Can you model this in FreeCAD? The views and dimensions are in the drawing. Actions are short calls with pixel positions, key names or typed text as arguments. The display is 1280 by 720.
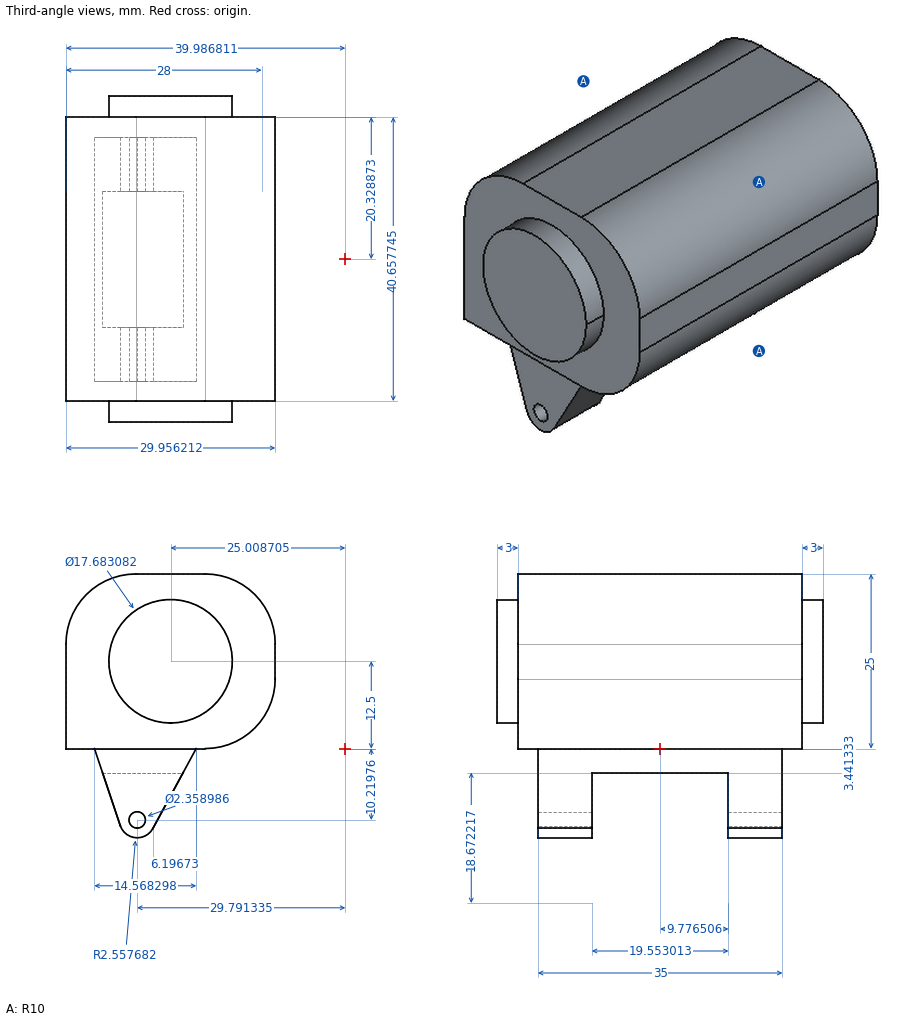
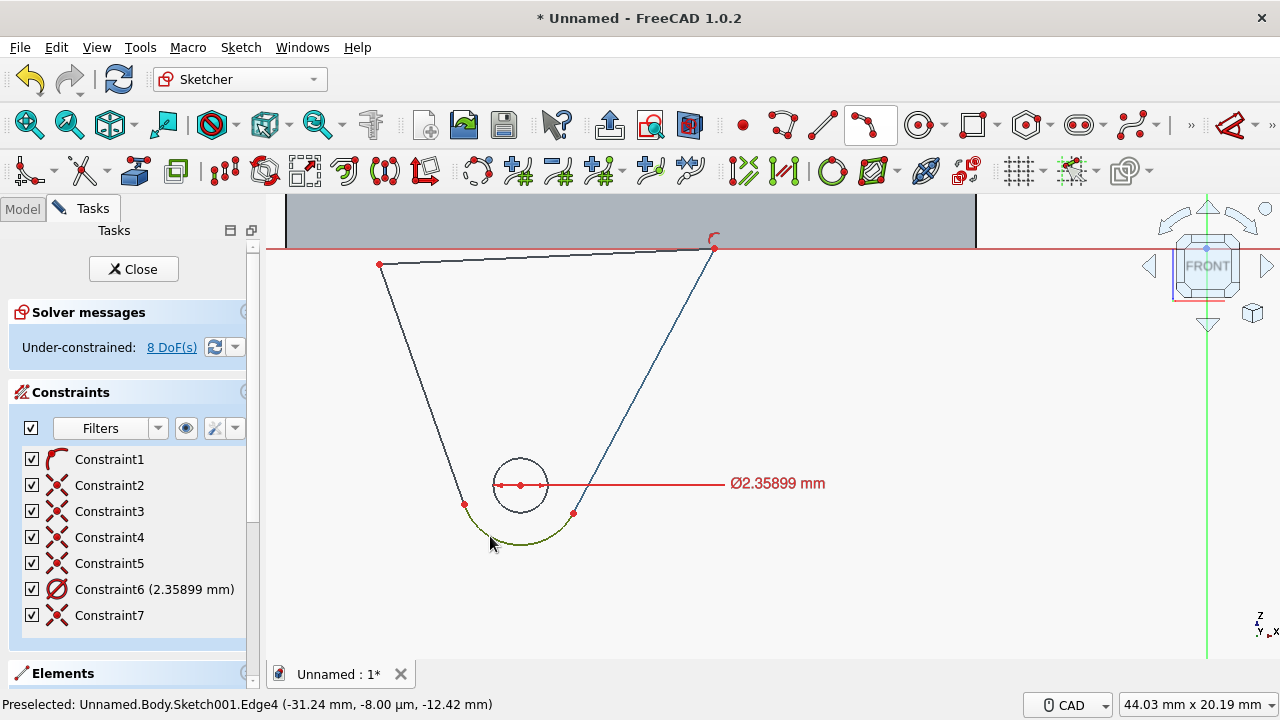
key(t)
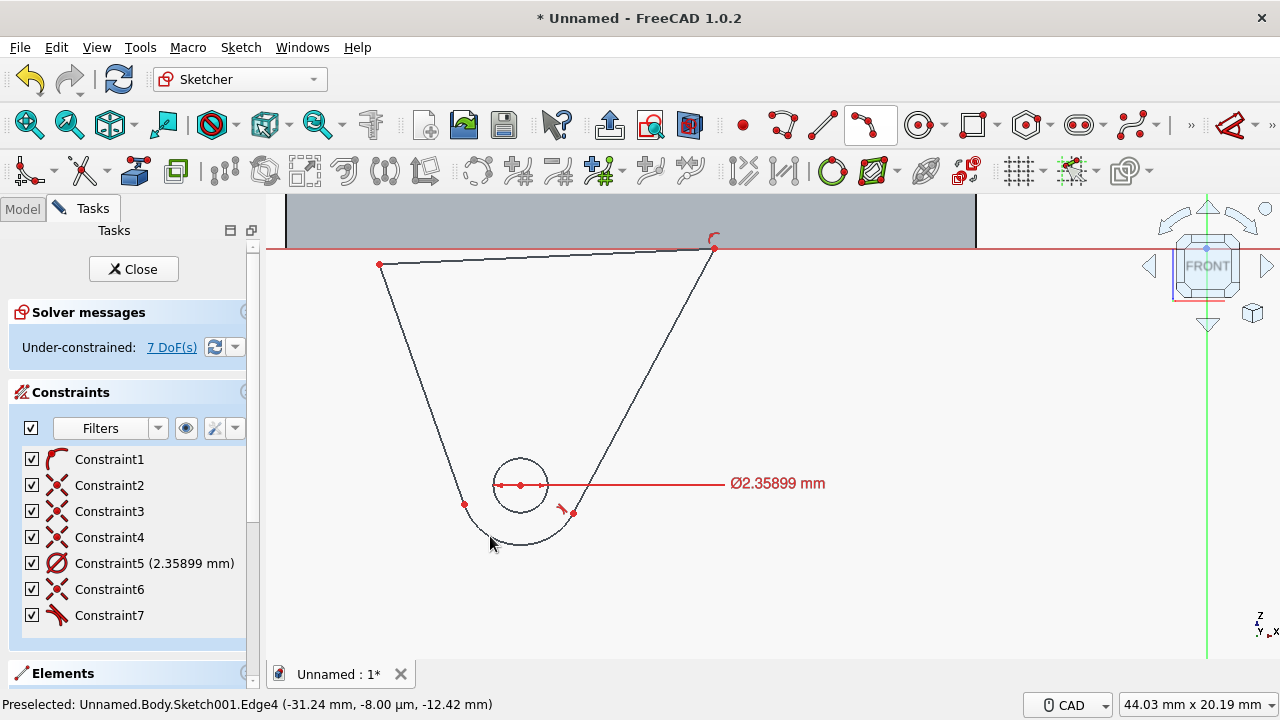
click(405, 336)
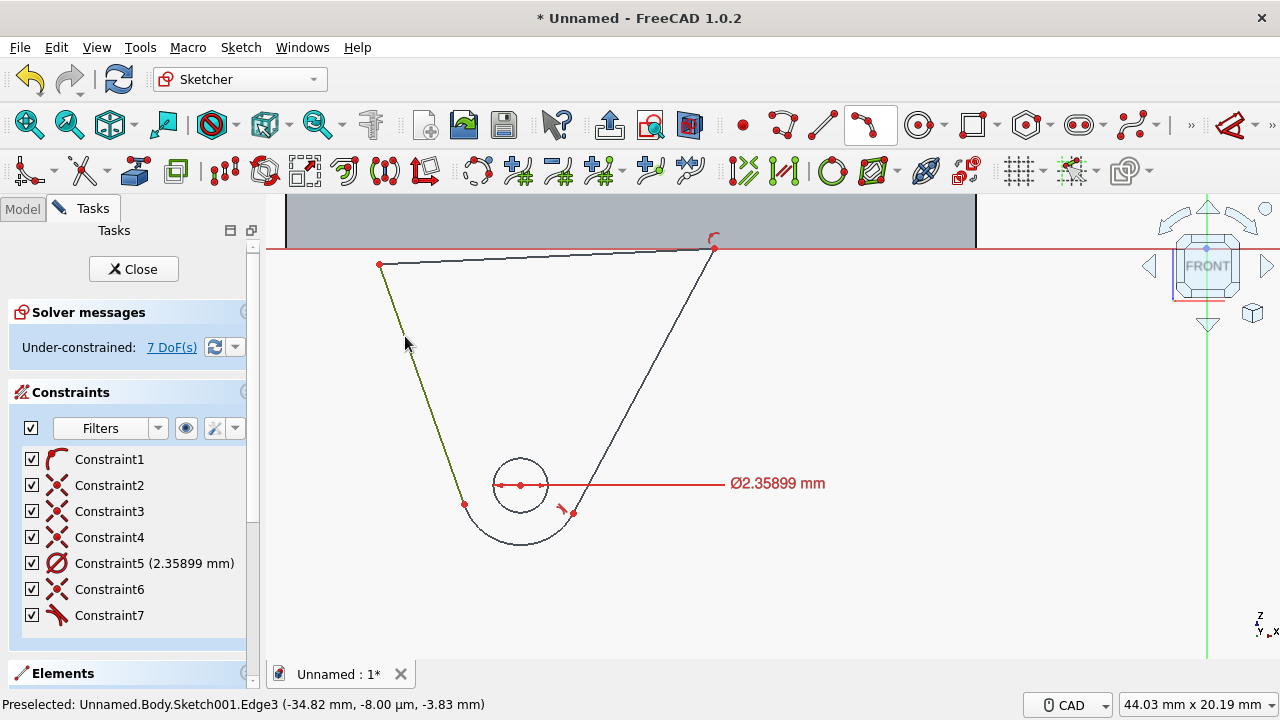
click(490, 536)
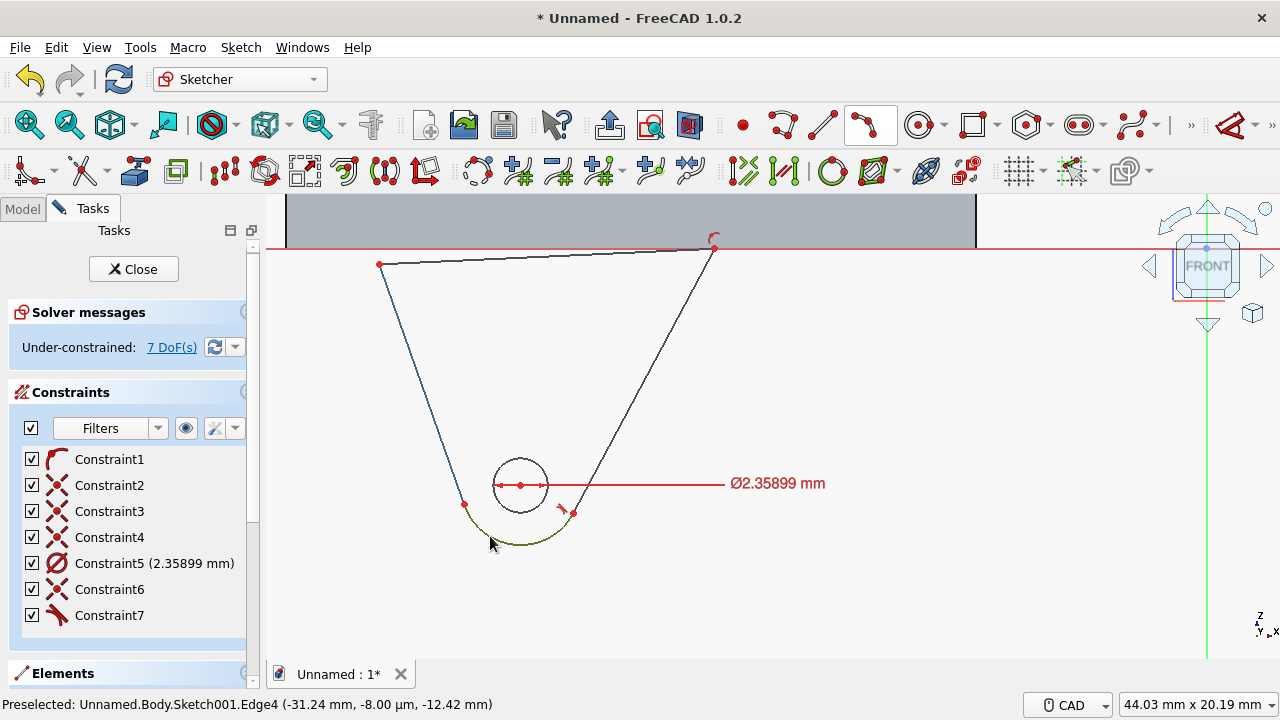
key(t)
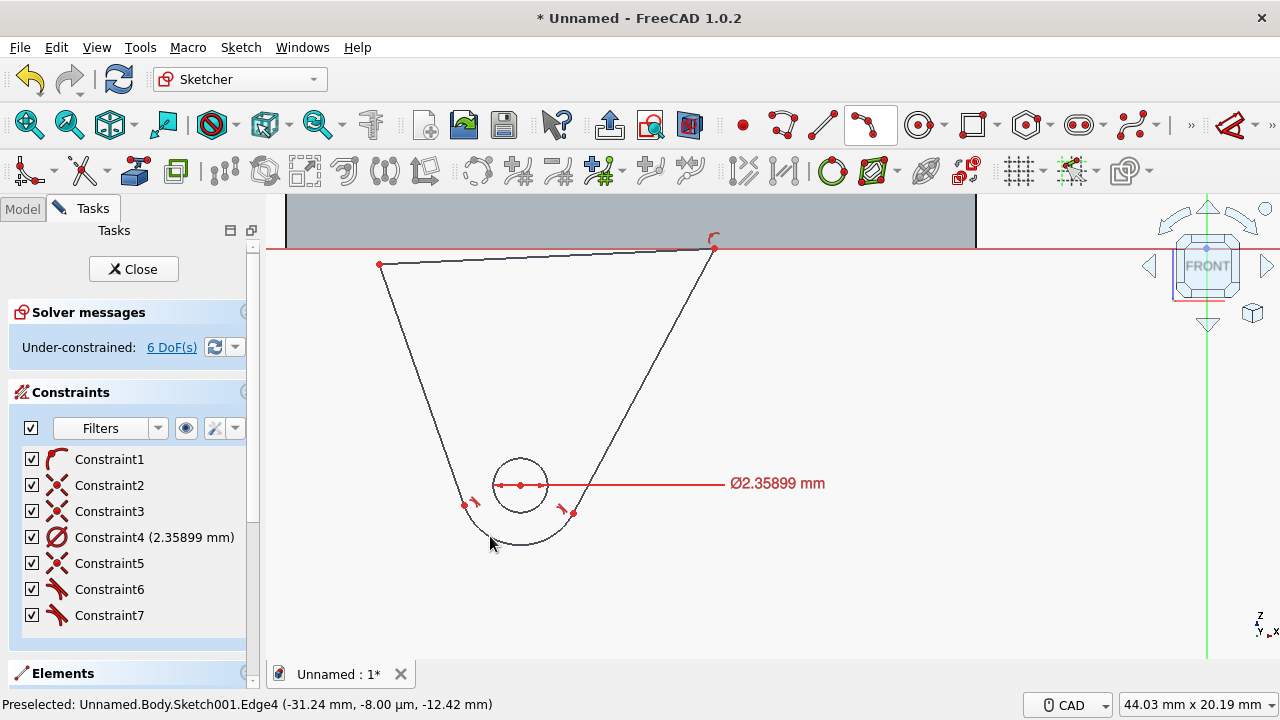
scroll(480, 260, up, 2)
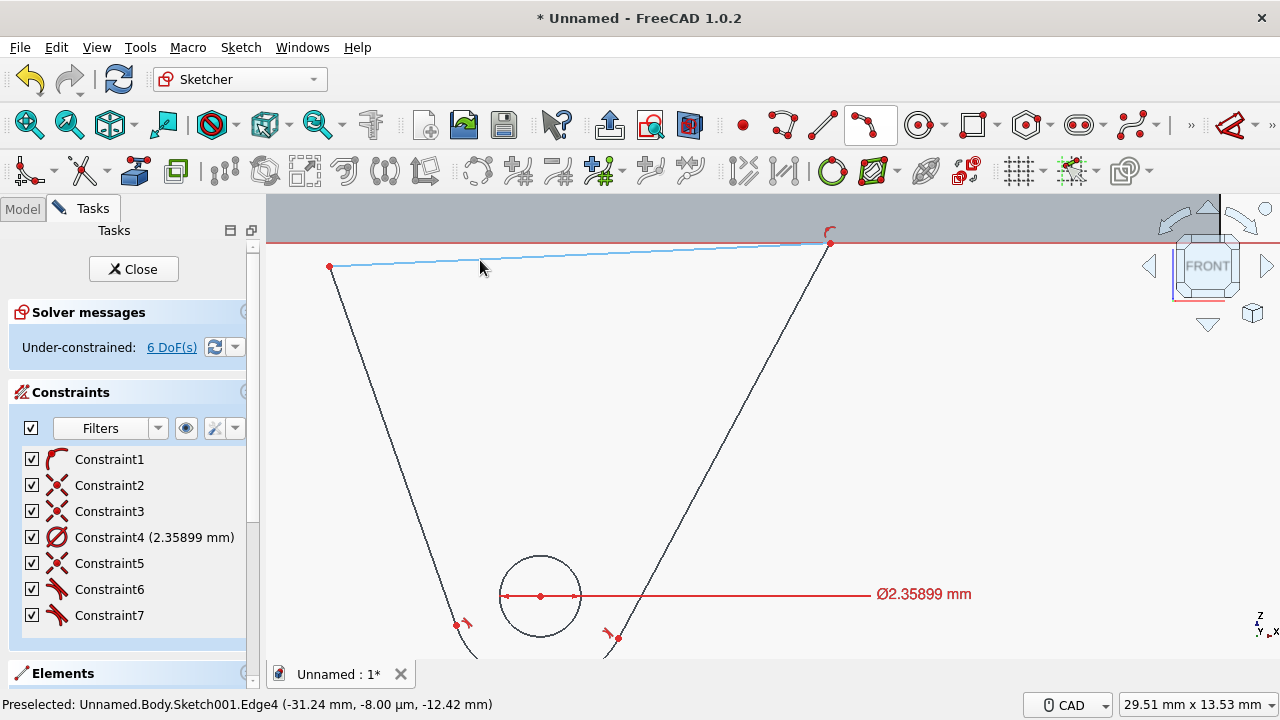
click(480, 259)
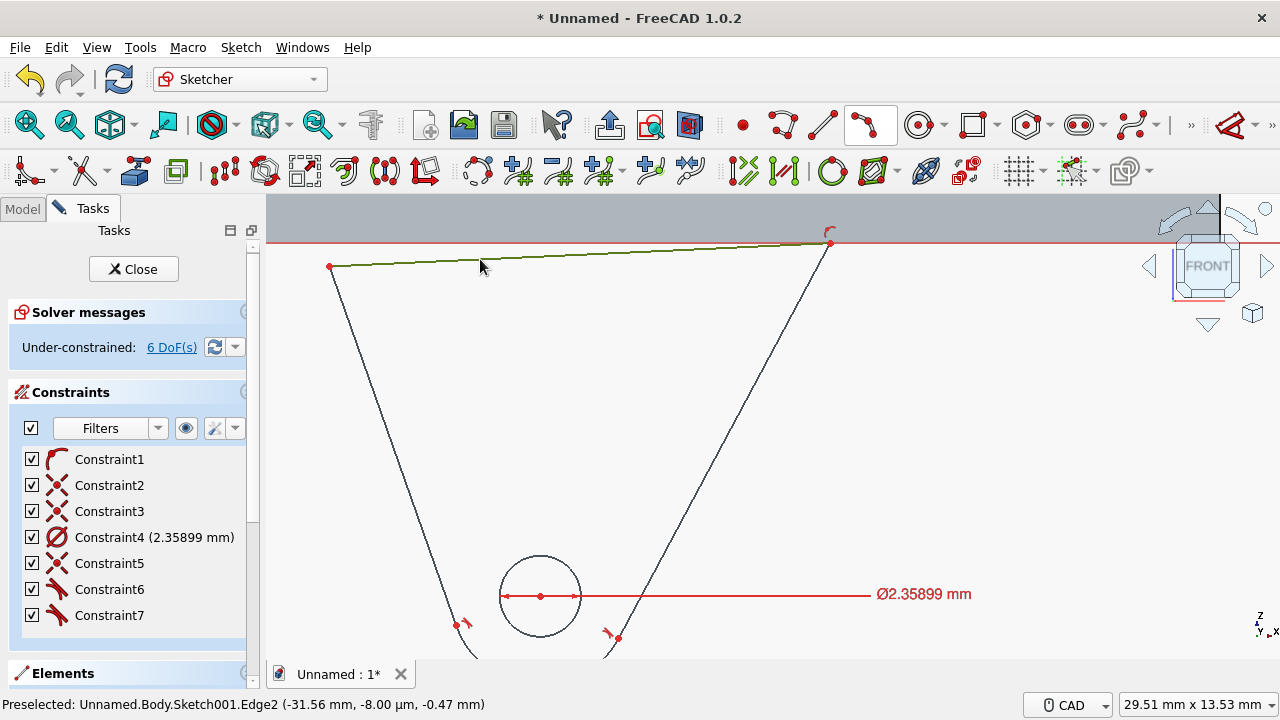
key(h)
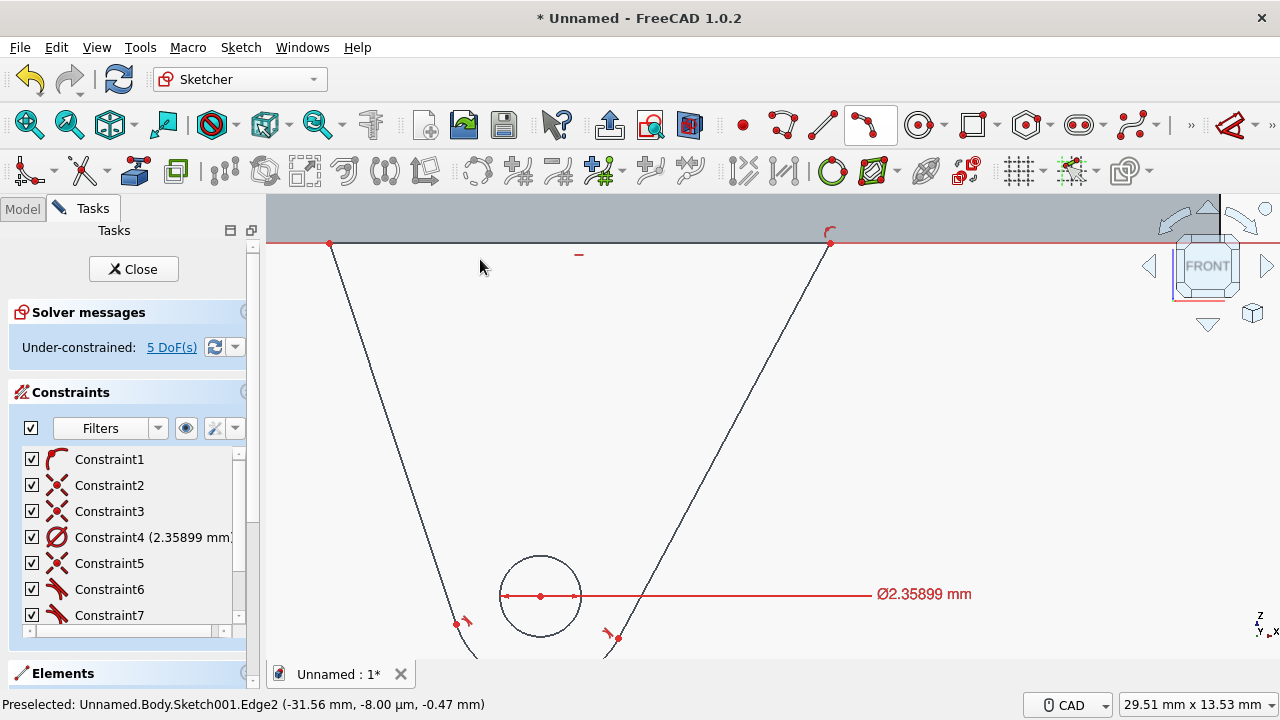
click(1230, 126)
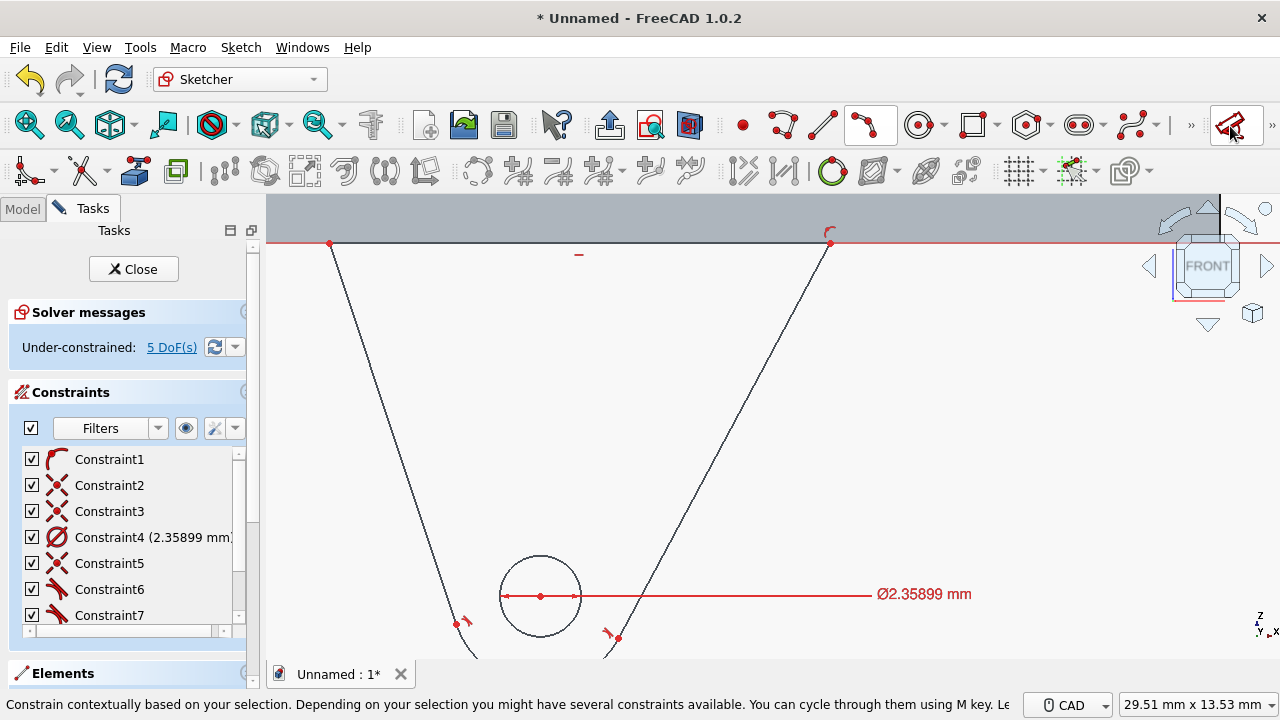
scroll(506, 397, down, 4)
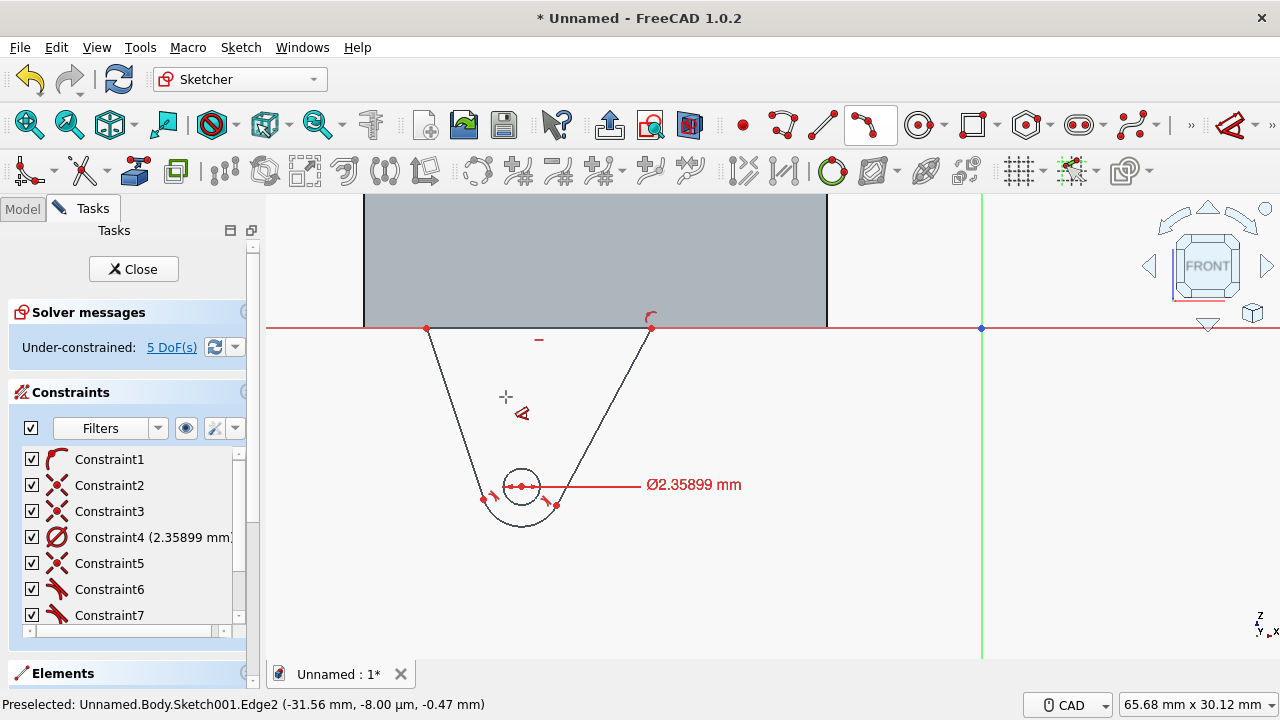
click(501, 521)
click(484, 548)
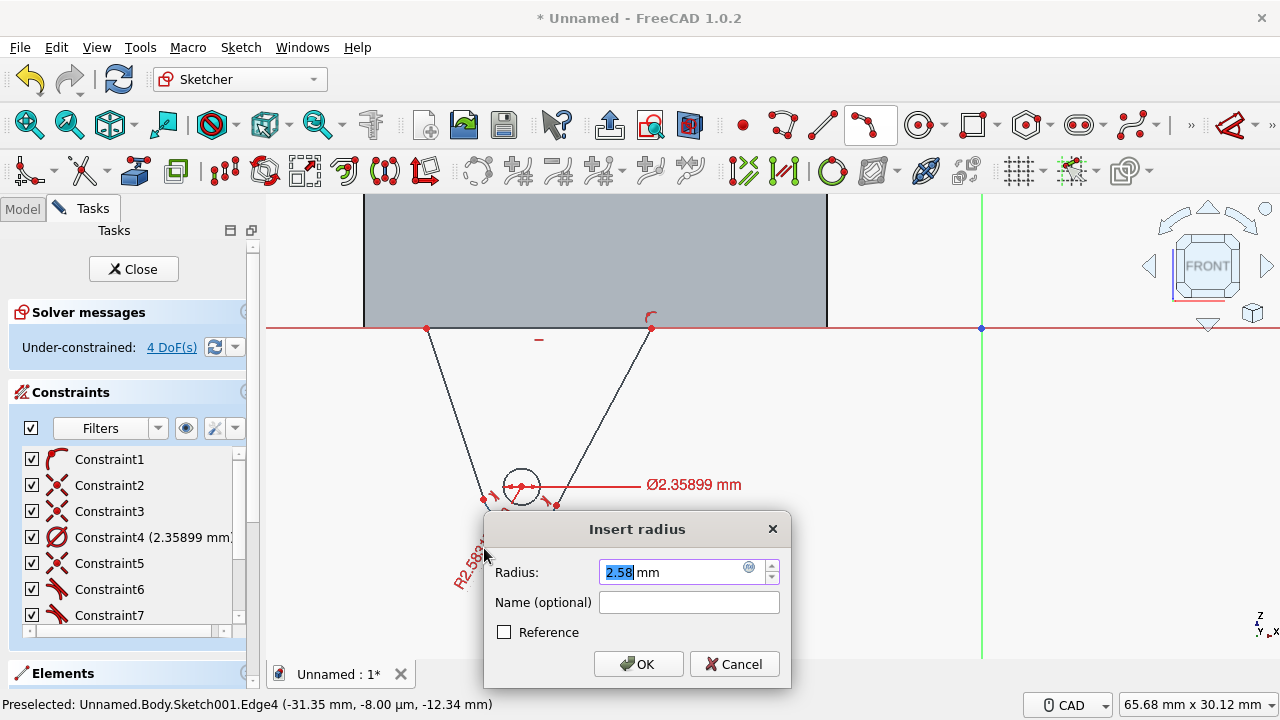
text(2.557682)
key(Return)